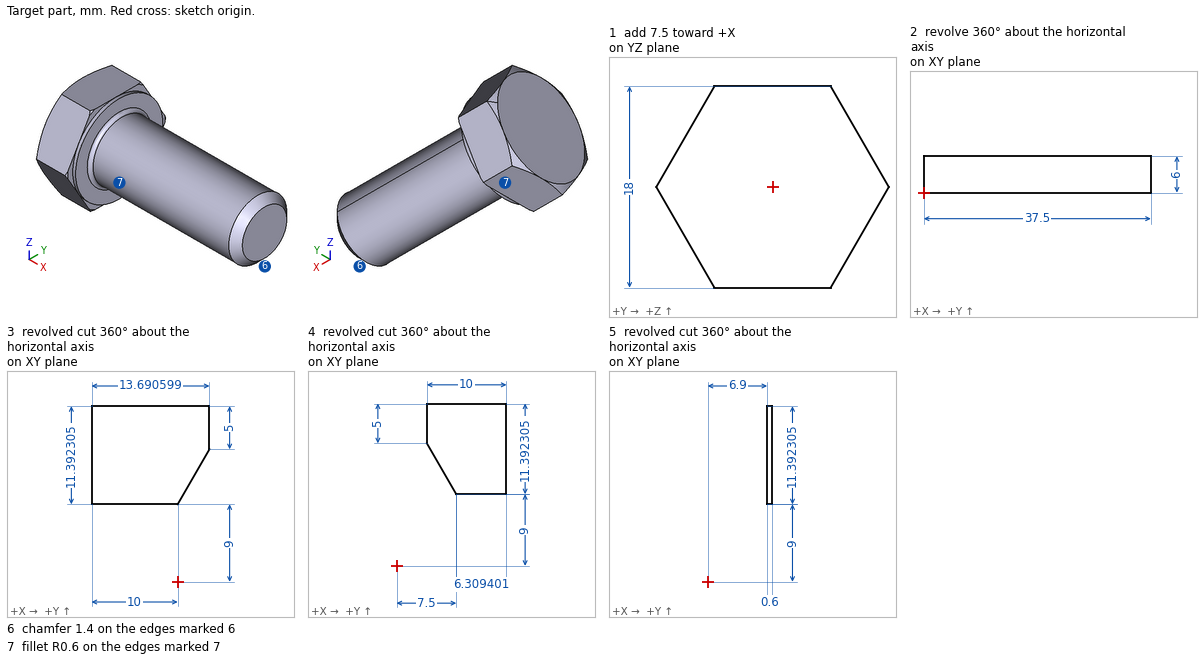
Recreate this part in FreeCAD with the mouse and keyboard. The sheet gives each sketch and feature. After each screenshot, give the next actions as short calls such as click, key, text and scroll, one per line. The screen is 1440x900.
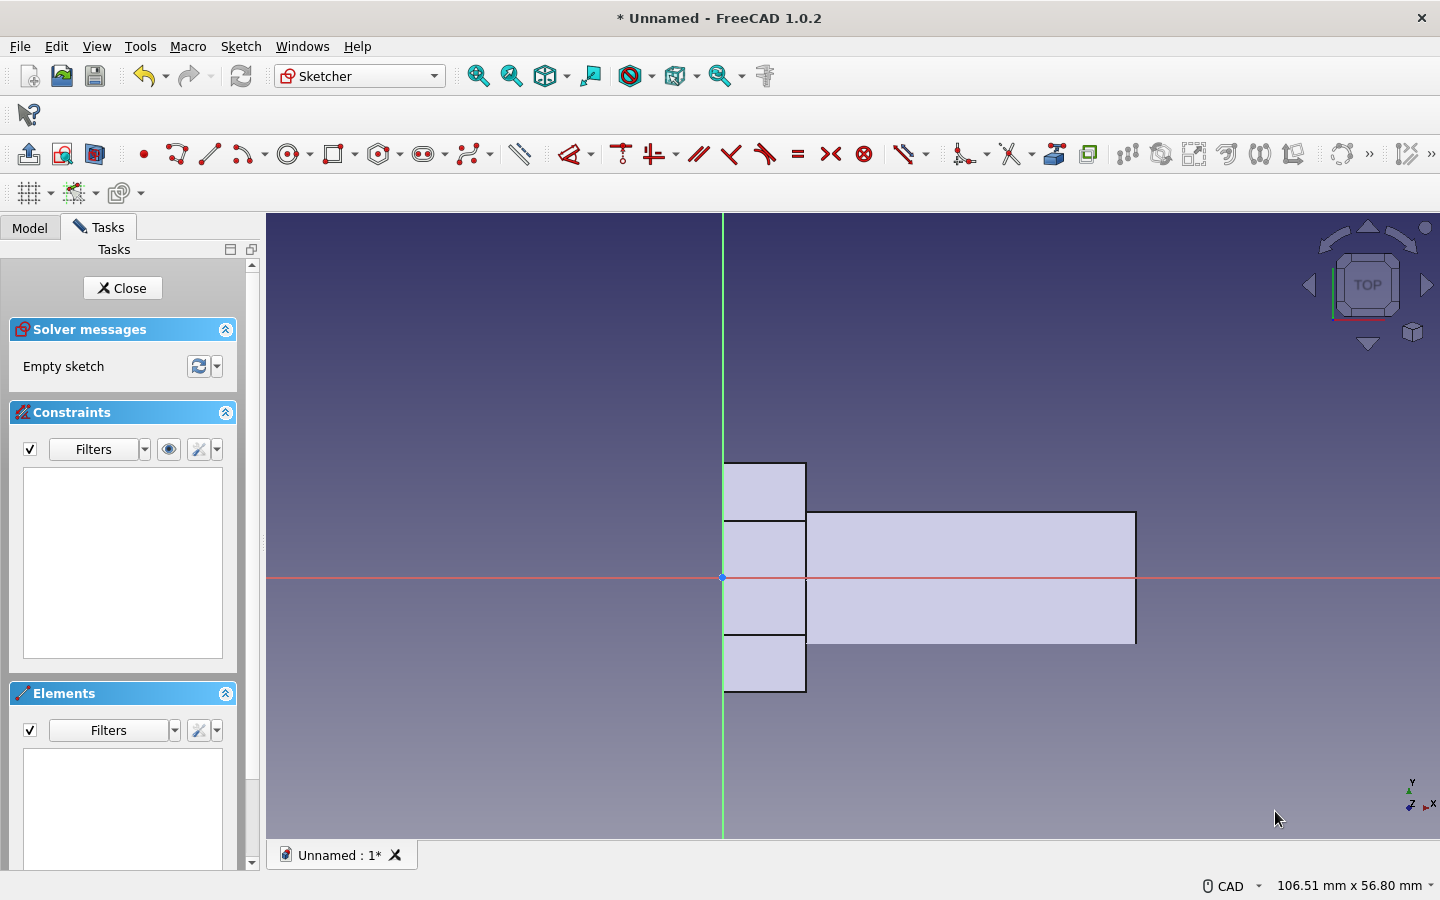
scroll(571, 392, up, 3)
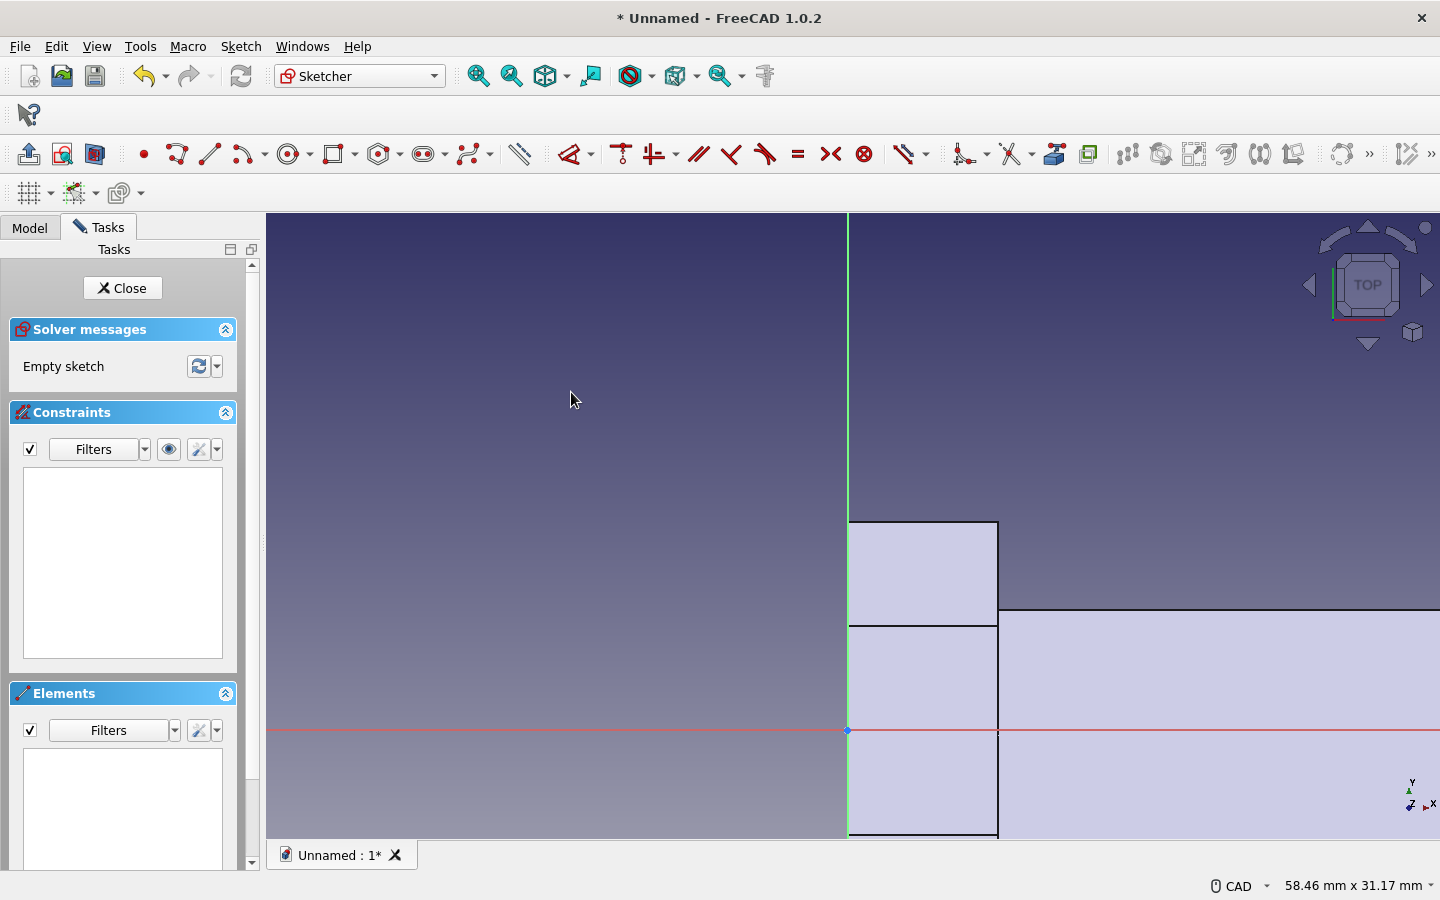
key(g)
key(m)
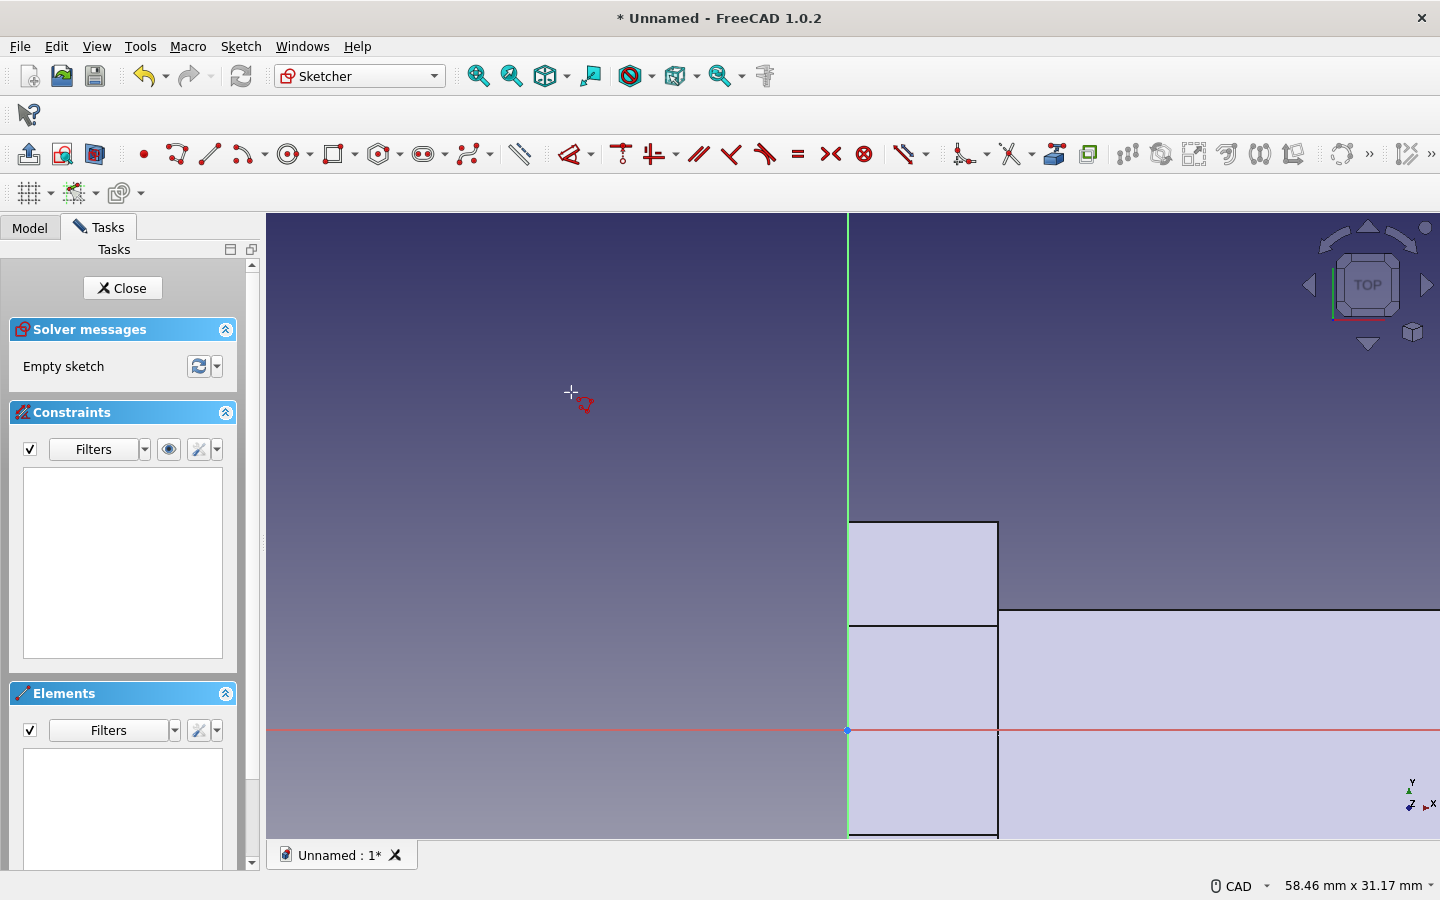
click(848, 550)
click(922, 421)
click(922, 321)
click(647, 321)
click(647, 550)
click(848, 551)
key(Escape)
key(Escape)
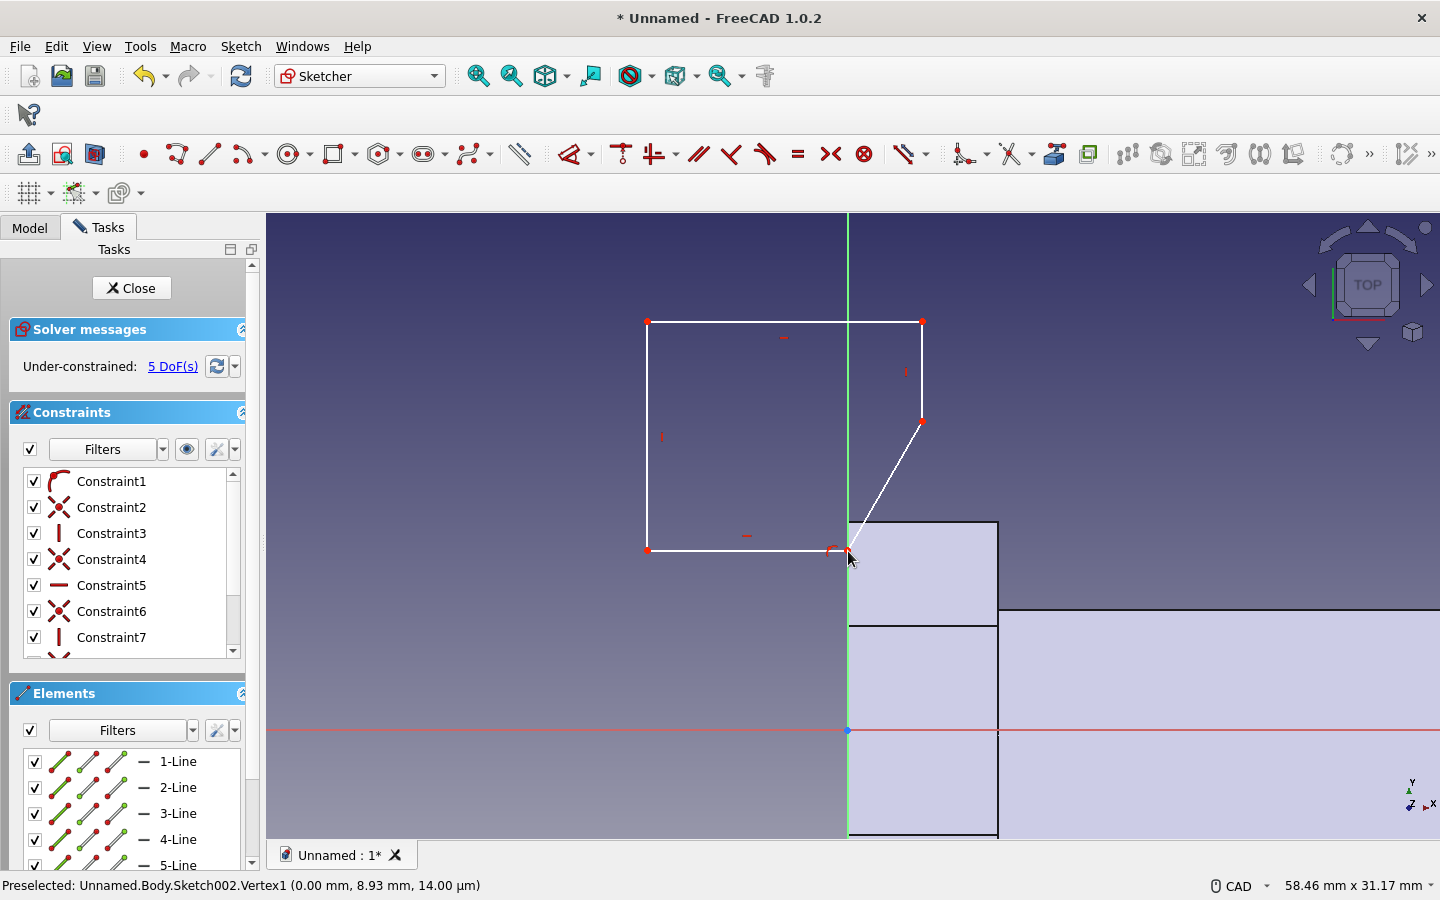
key(d)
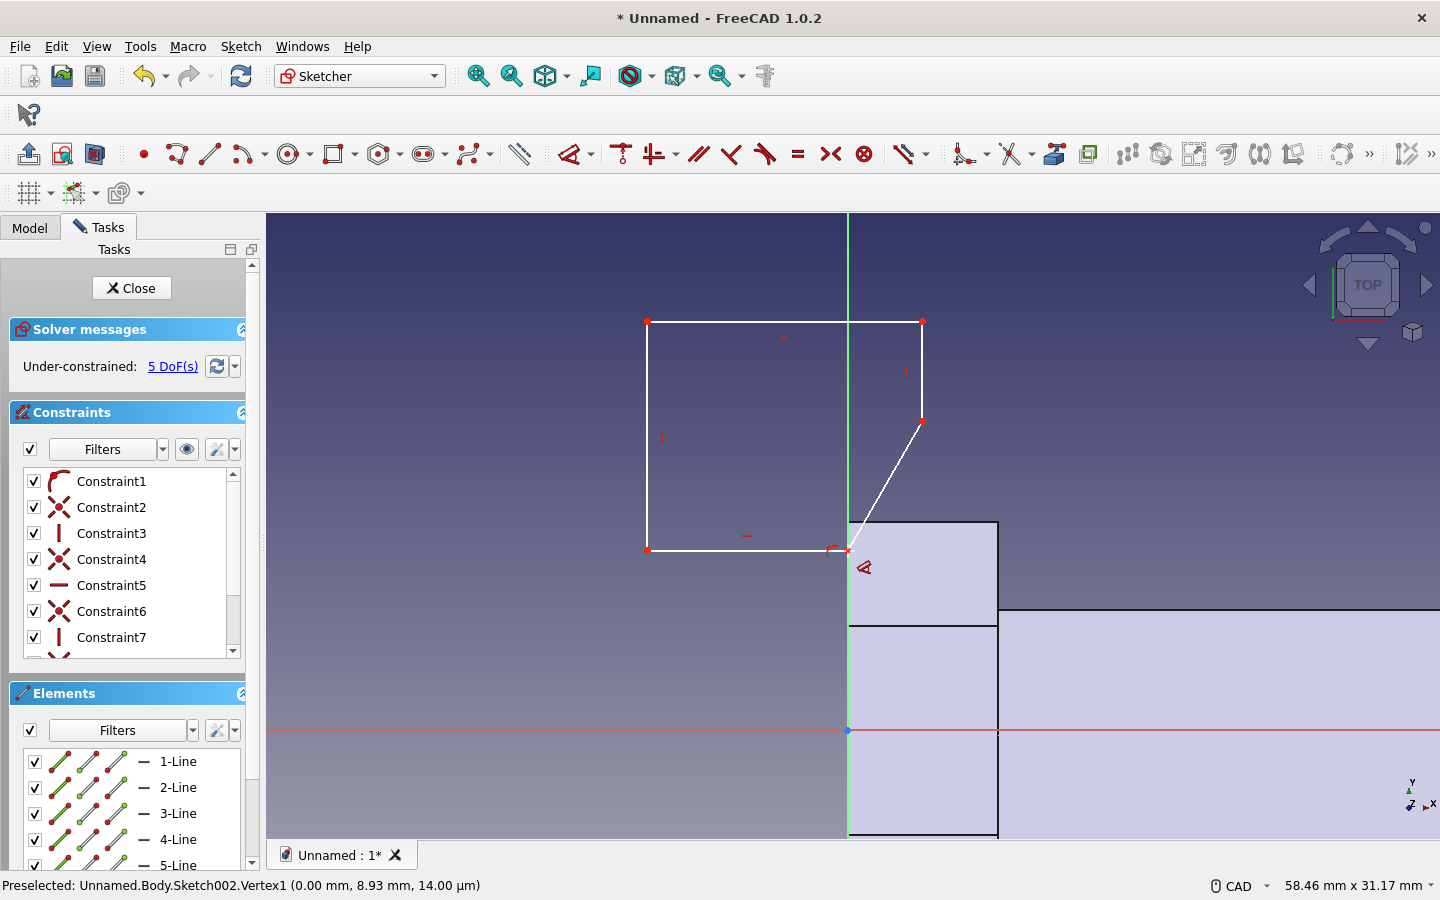
click(922, 392)
click(956, 372)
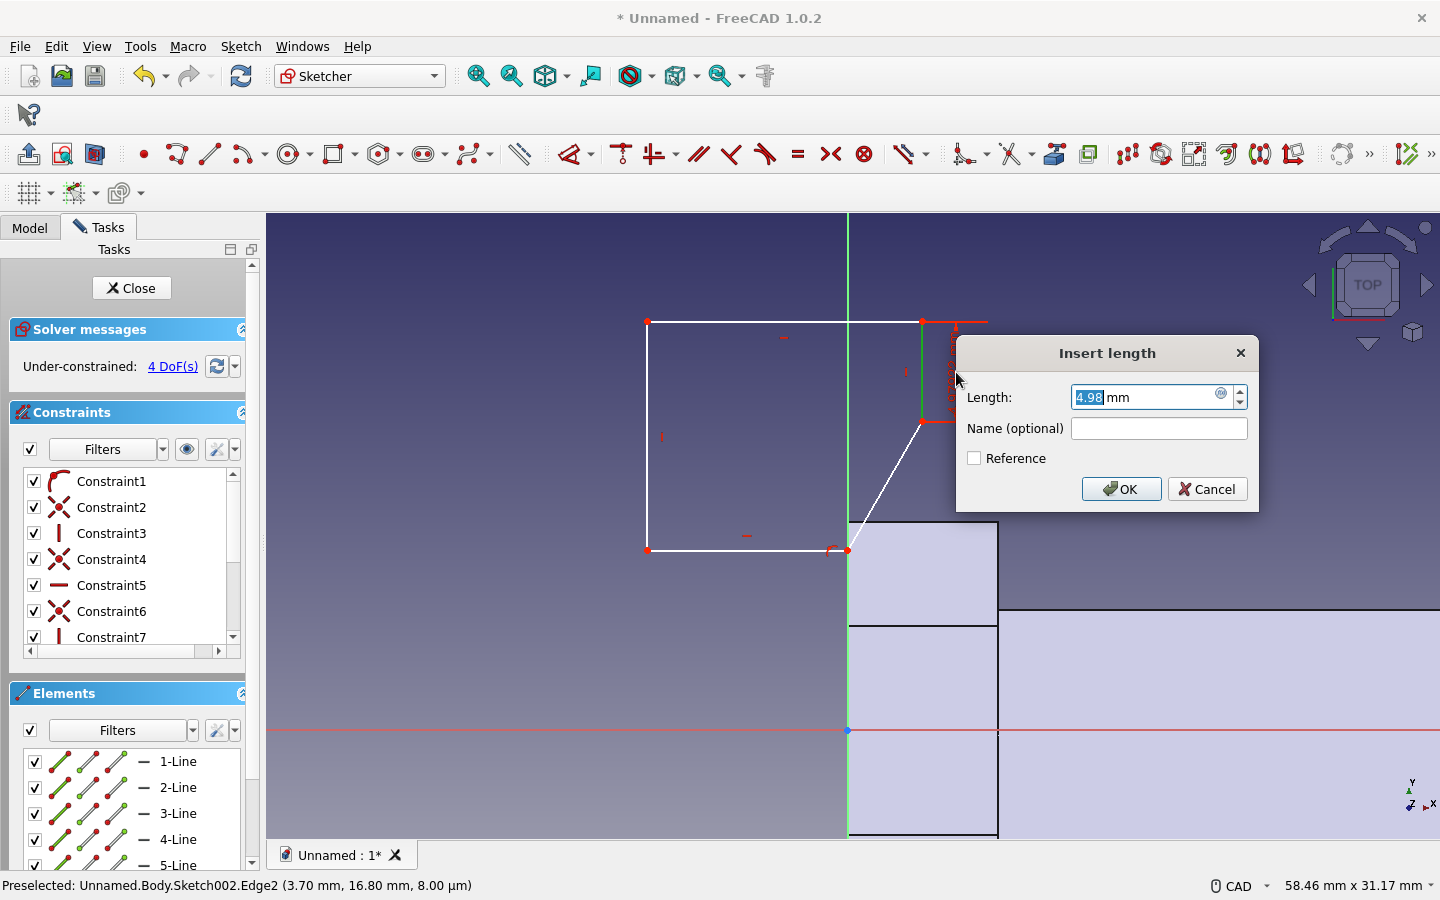
text(5)
key(Return)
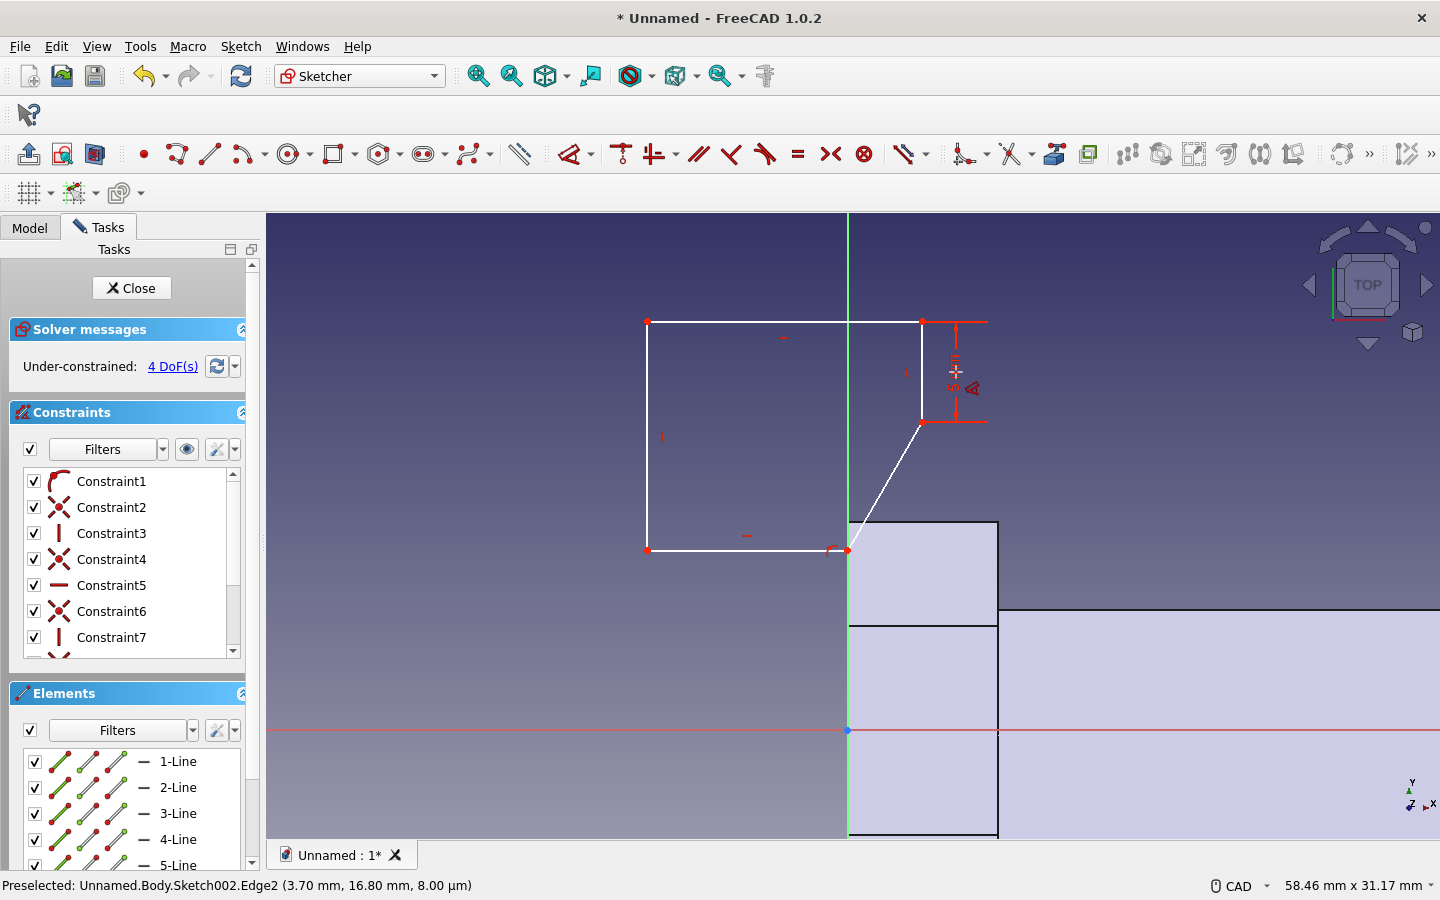
click(707, 551)
click(747, 585)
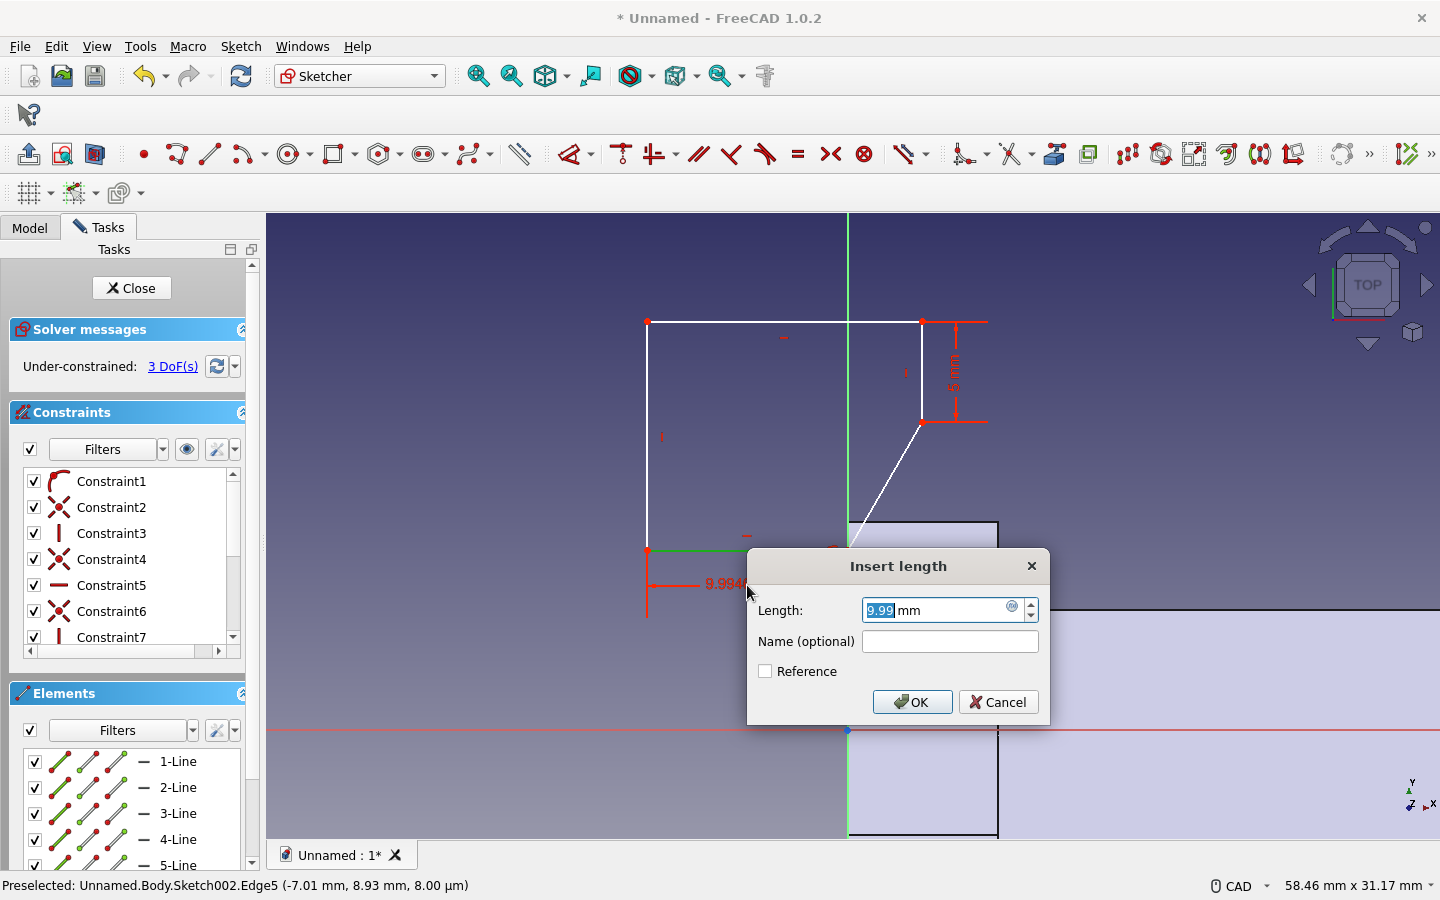
text(10)
key(Return)